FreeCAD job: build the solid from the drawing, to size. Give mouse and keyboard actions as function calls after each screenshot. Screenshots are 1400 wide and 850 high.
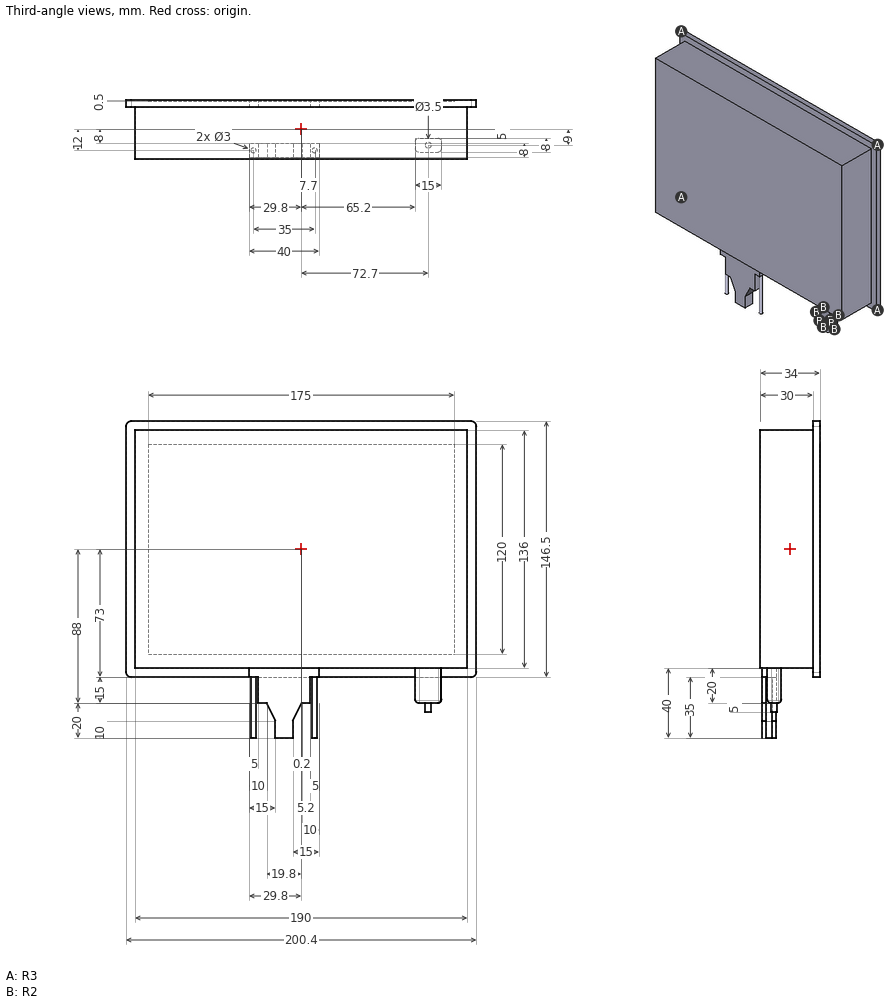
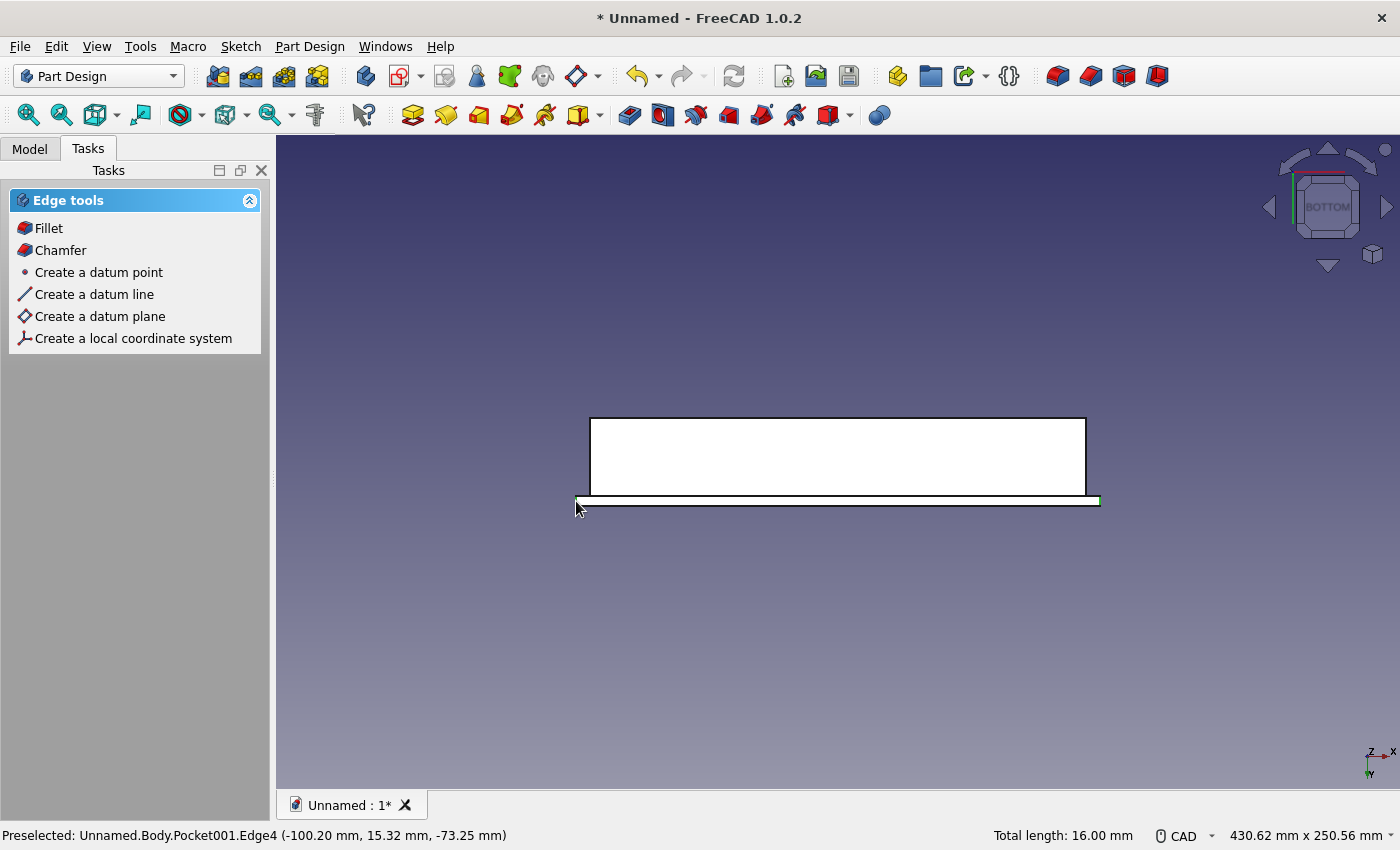
click(1058, 76)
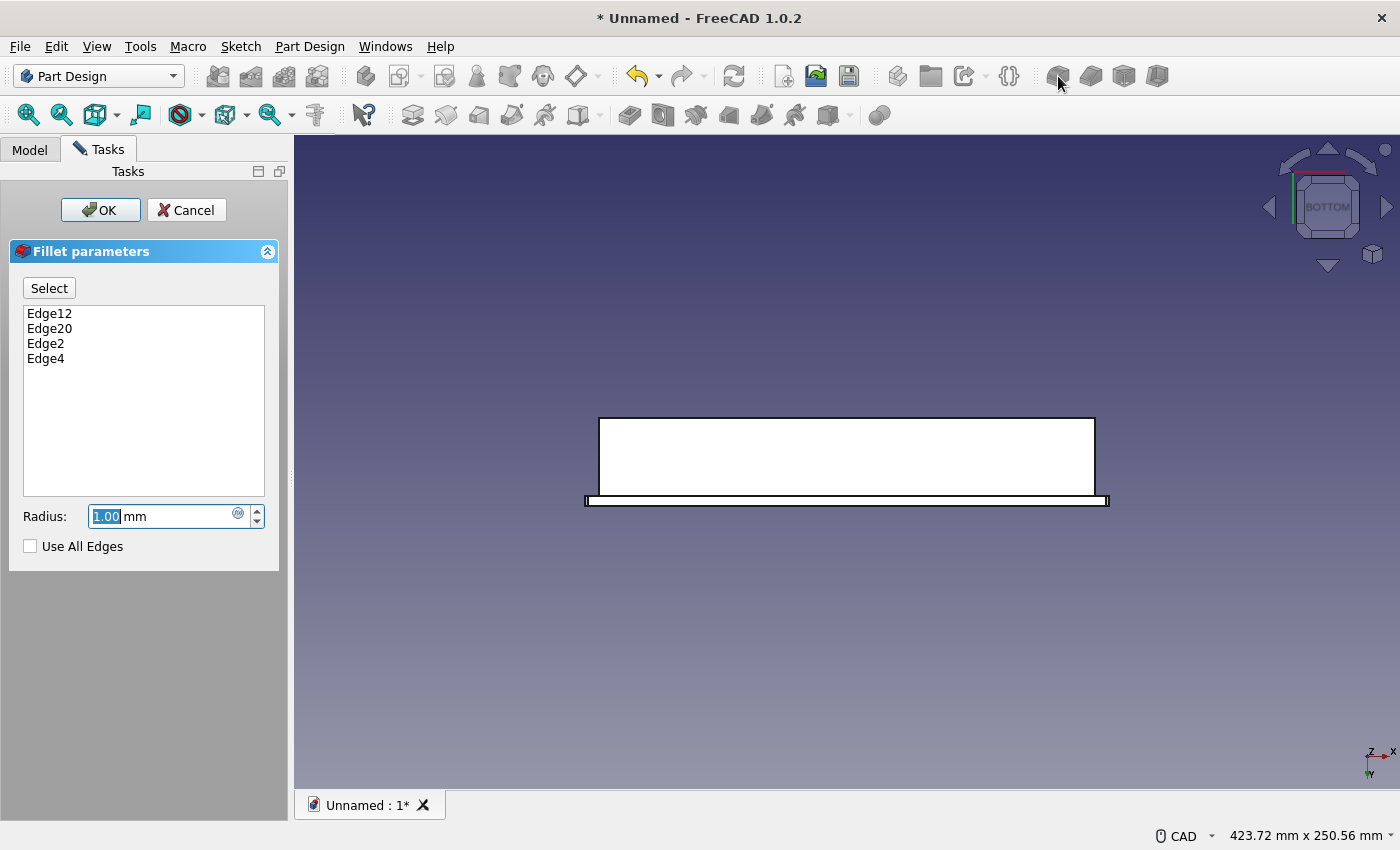
text(3)
key(Tab)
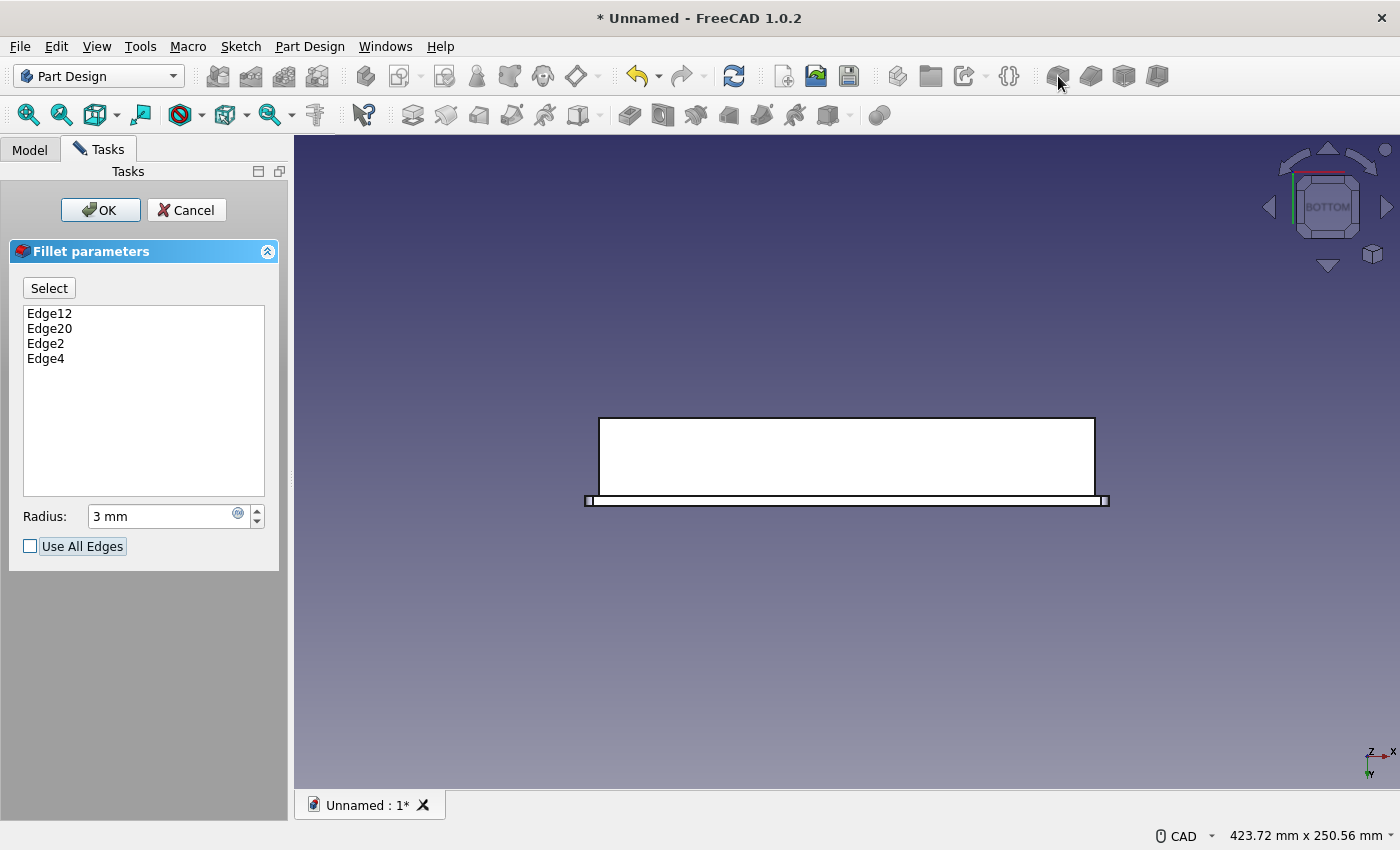
click(101, 210)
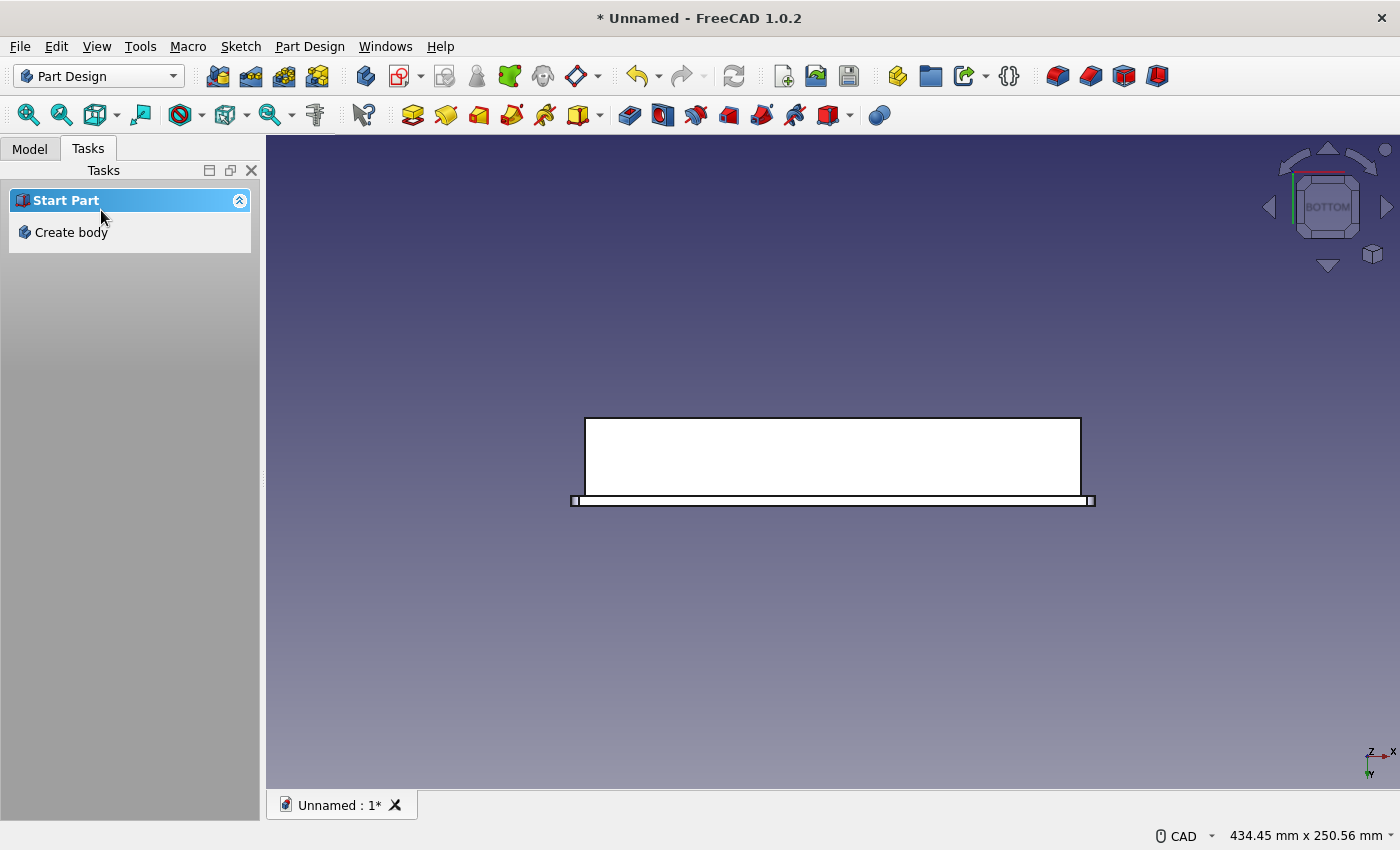
click(975, 456)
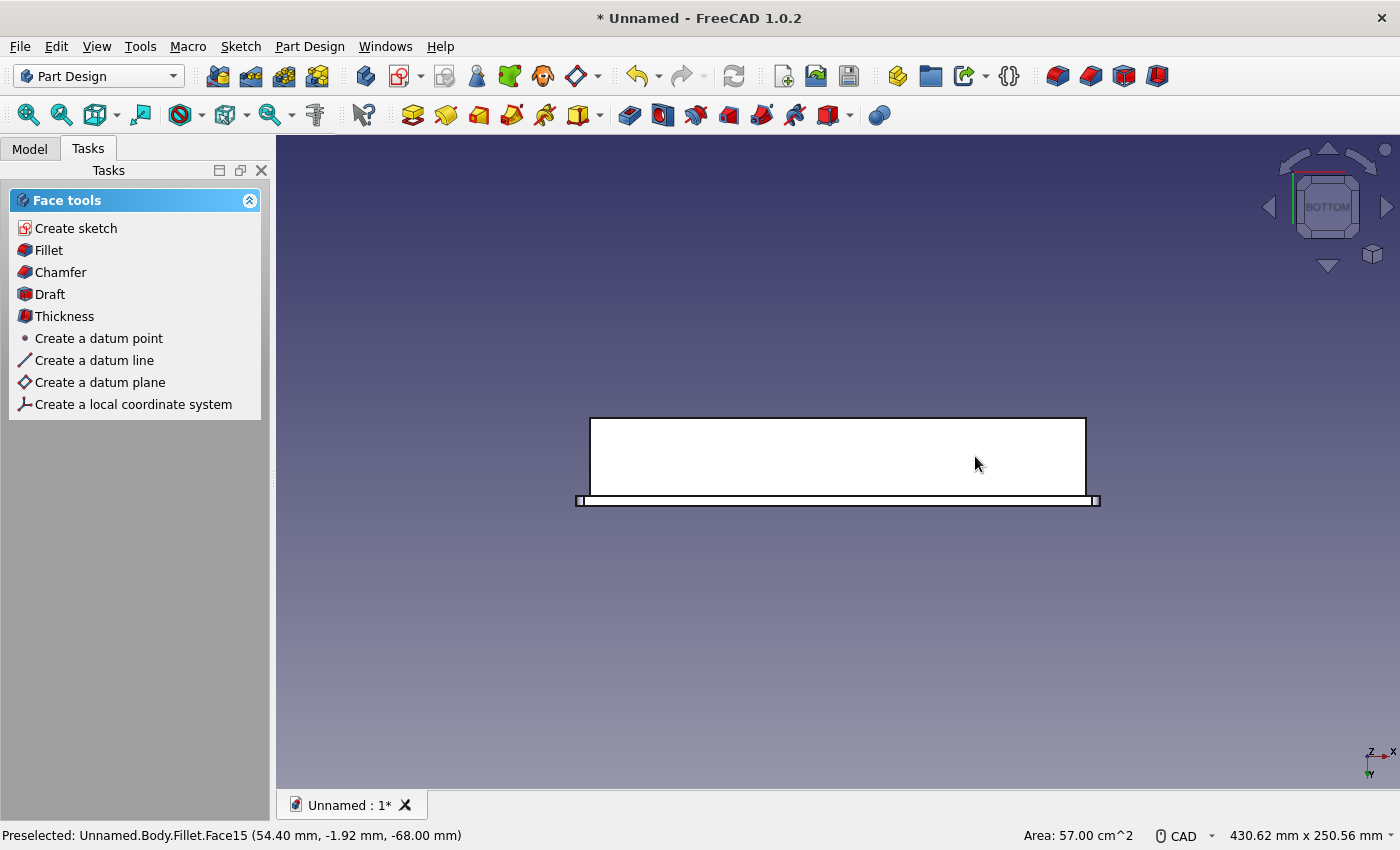
click(398, 76)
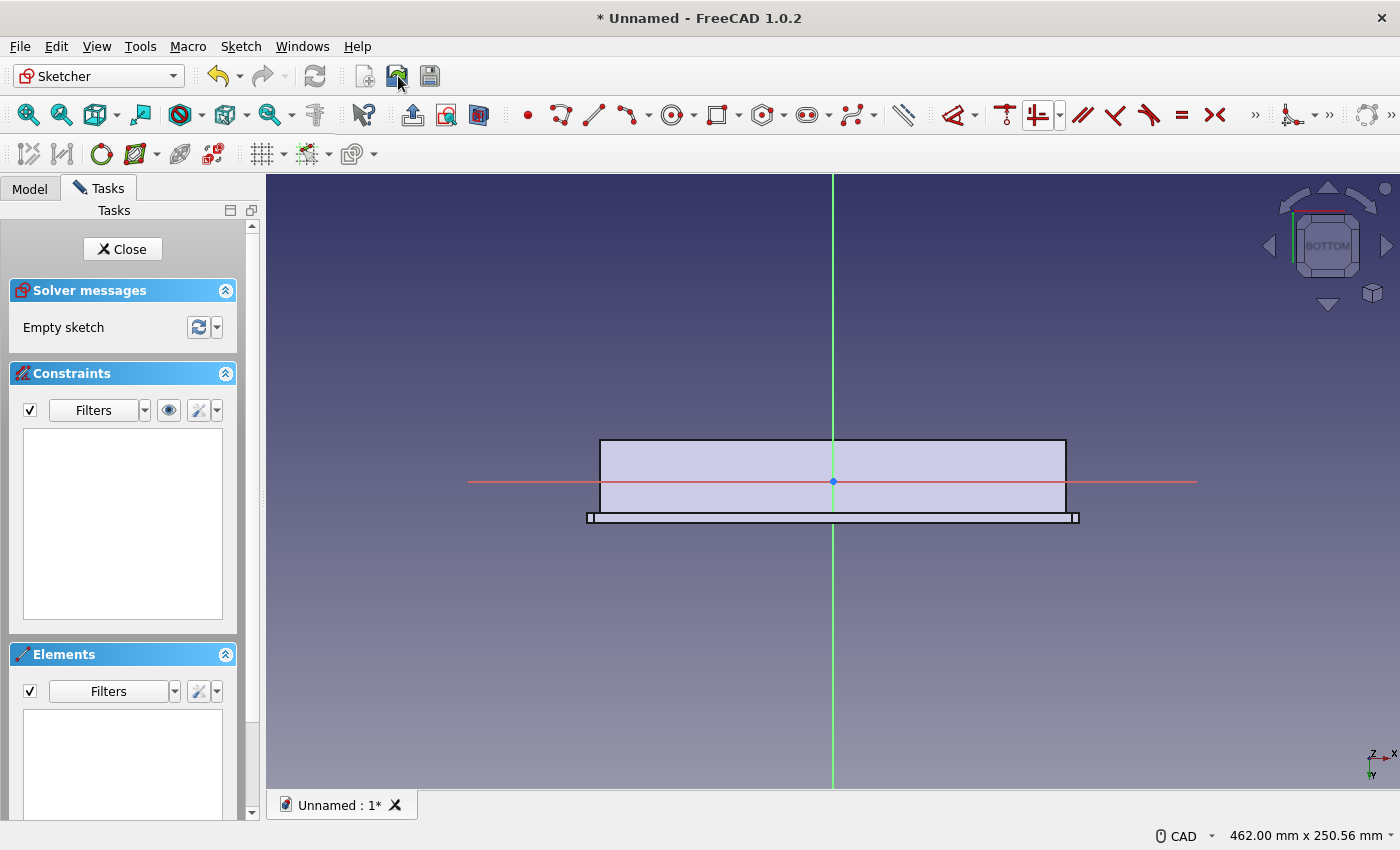
scroll(816, 459, up, 10)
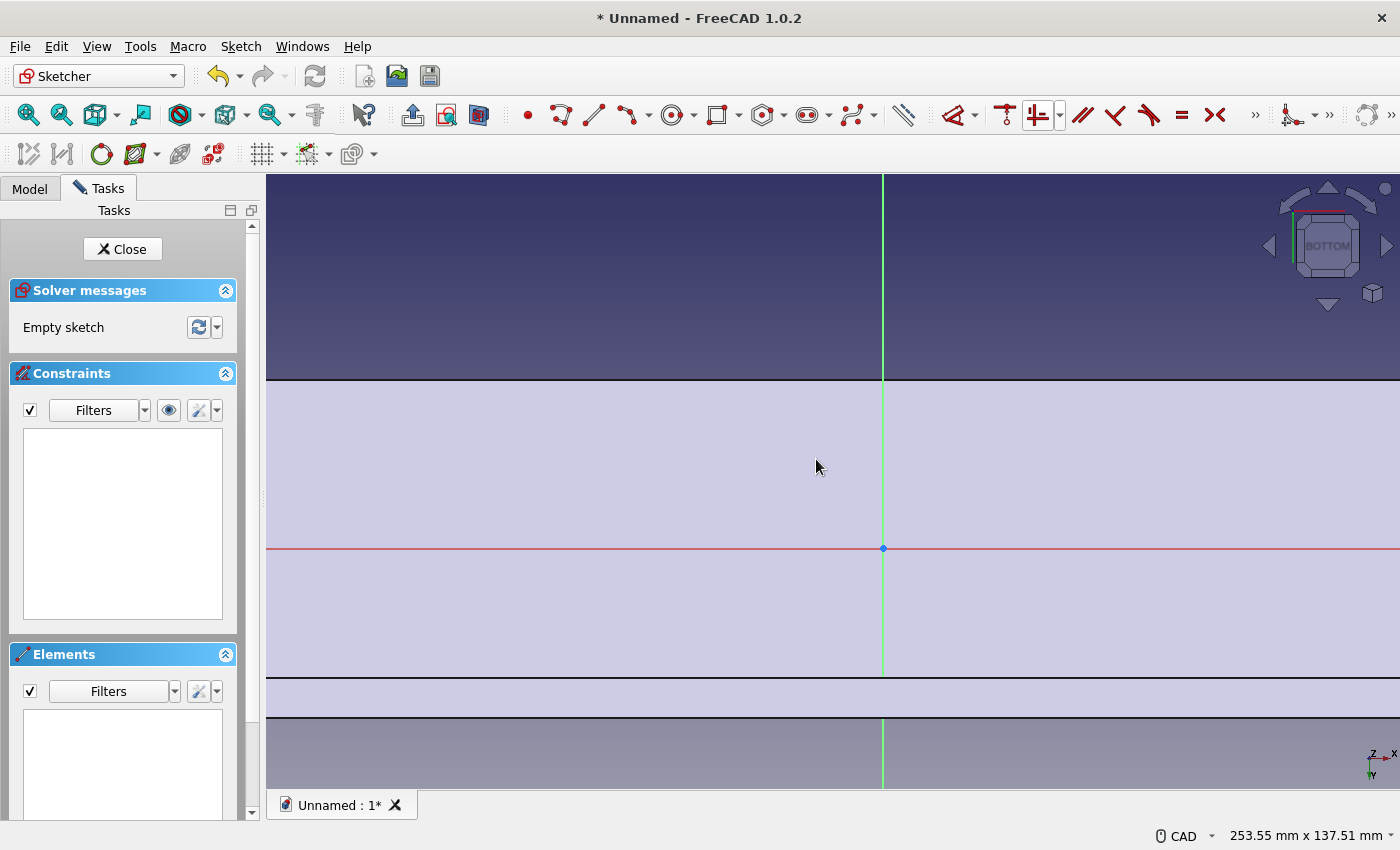
click(716, 116)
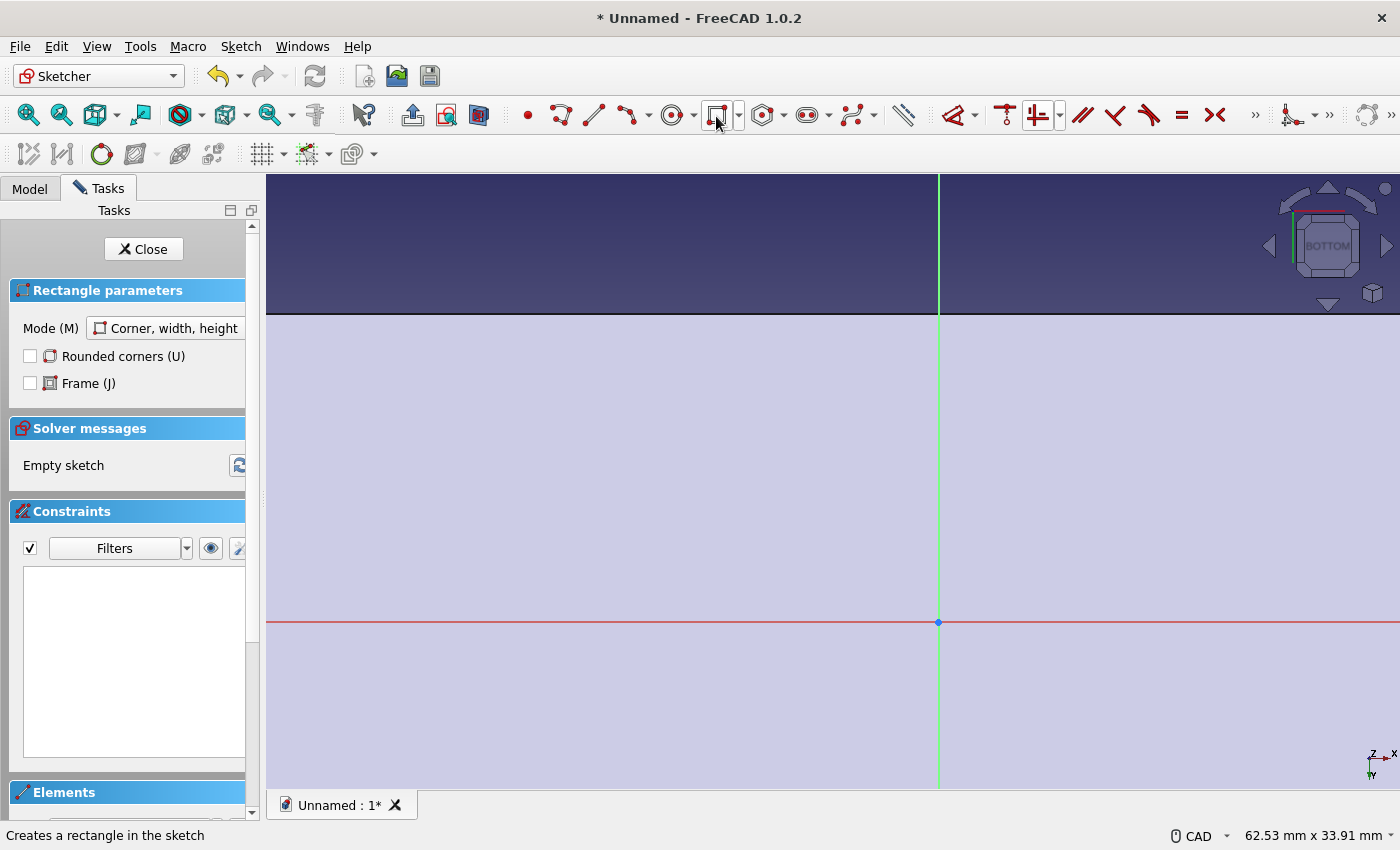
click(398, 332)
move(1124, 477)